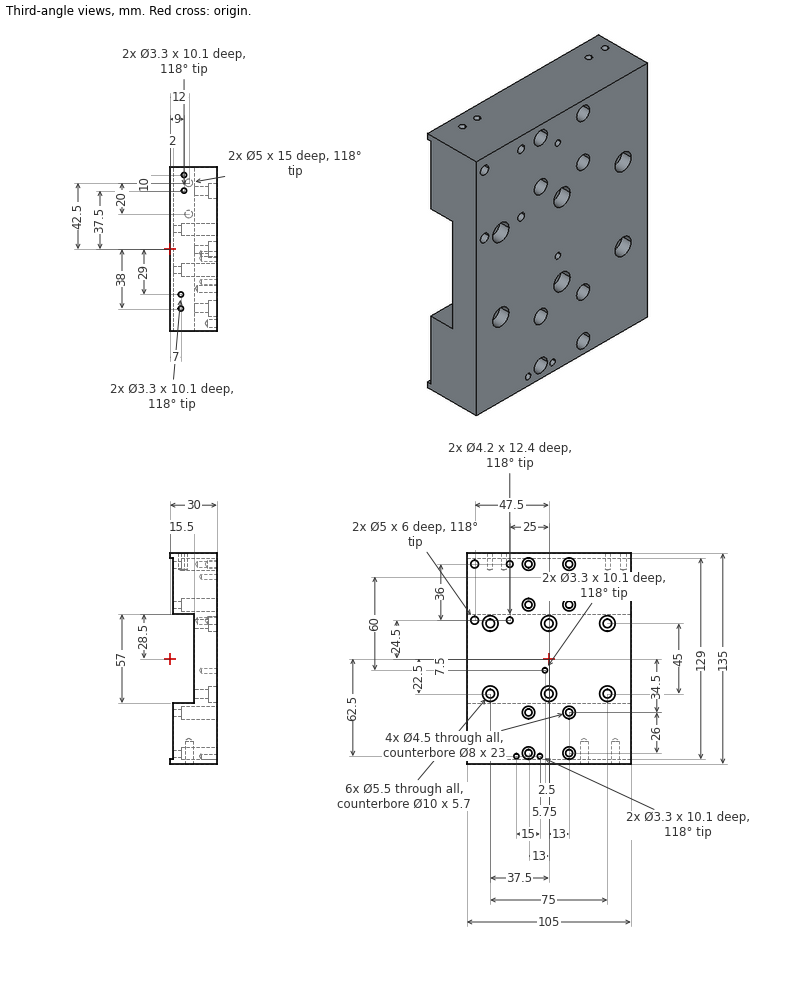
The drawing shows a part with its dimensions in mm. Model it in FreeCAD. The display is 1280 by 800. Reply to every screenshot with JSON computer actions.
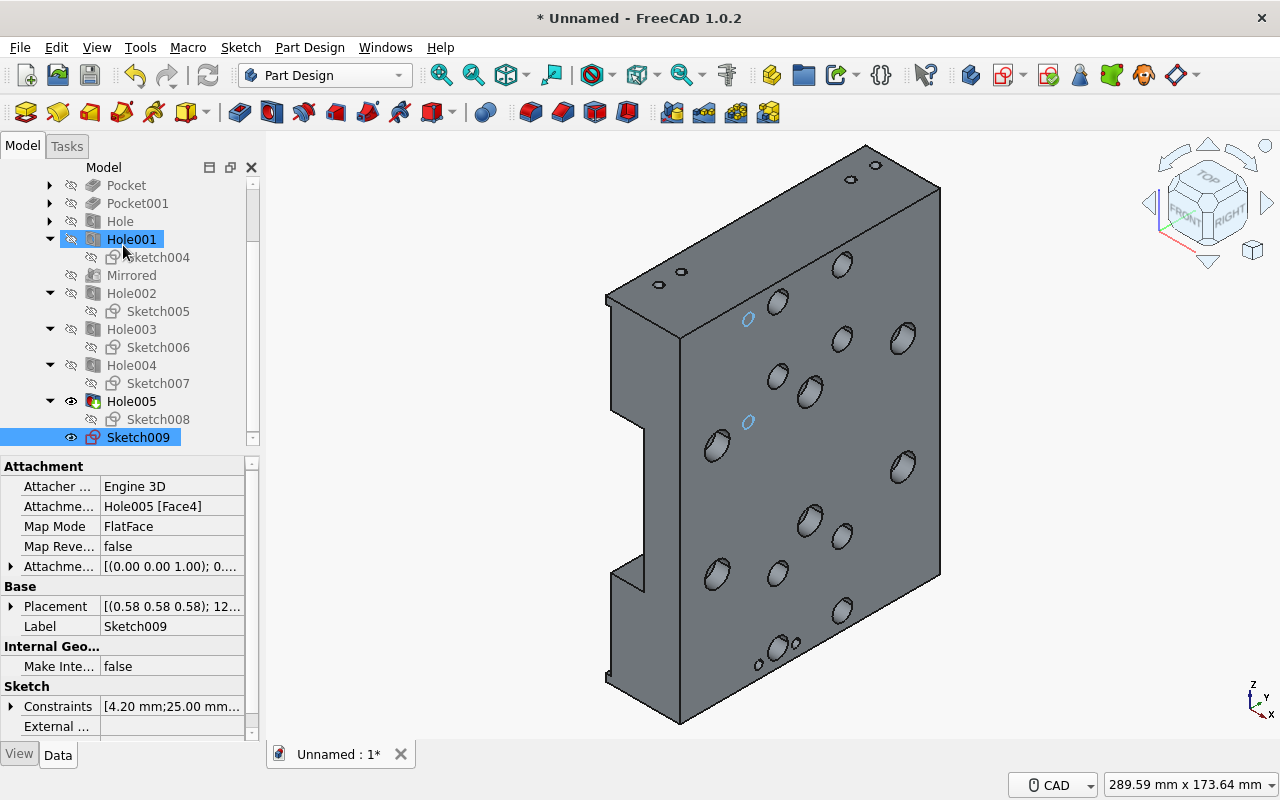
{"action": "left_click", "coordinate": [272, 112]}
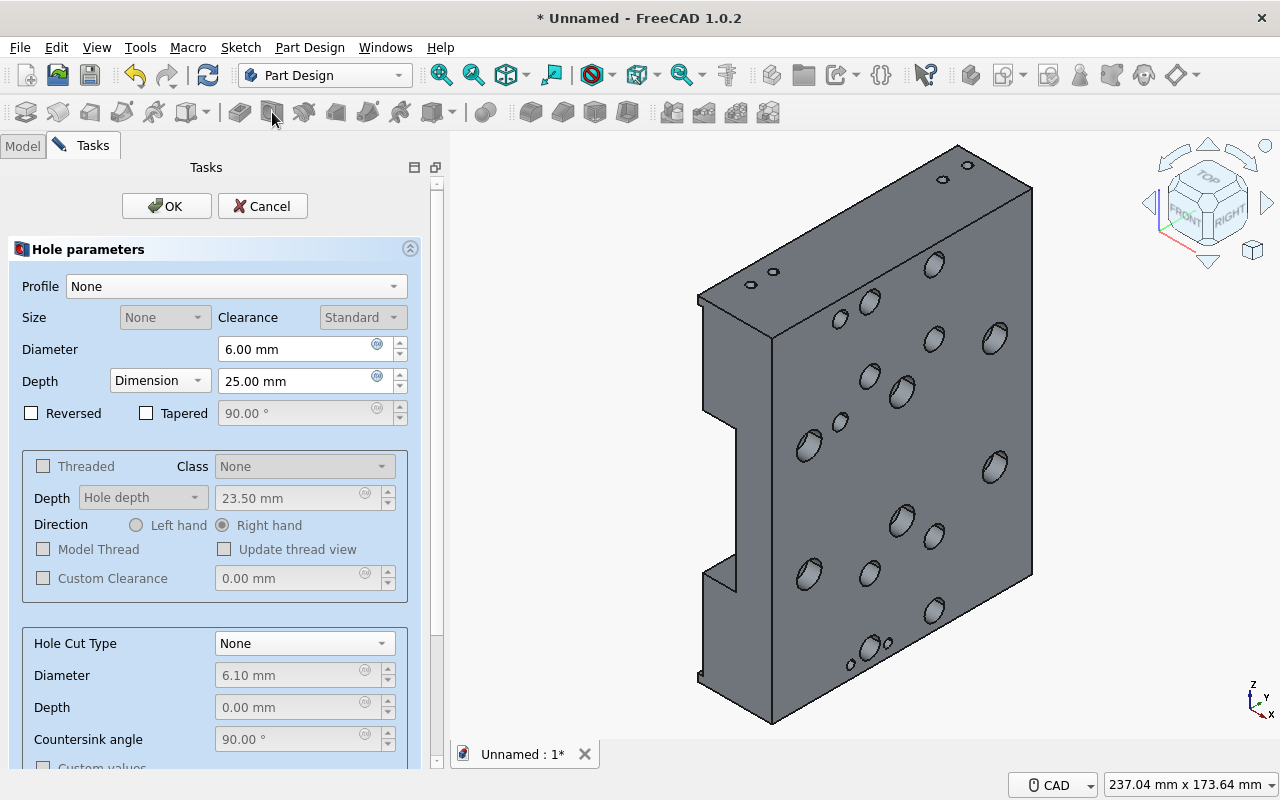
{"action": "triple_click", "coordinate": [305, 349]}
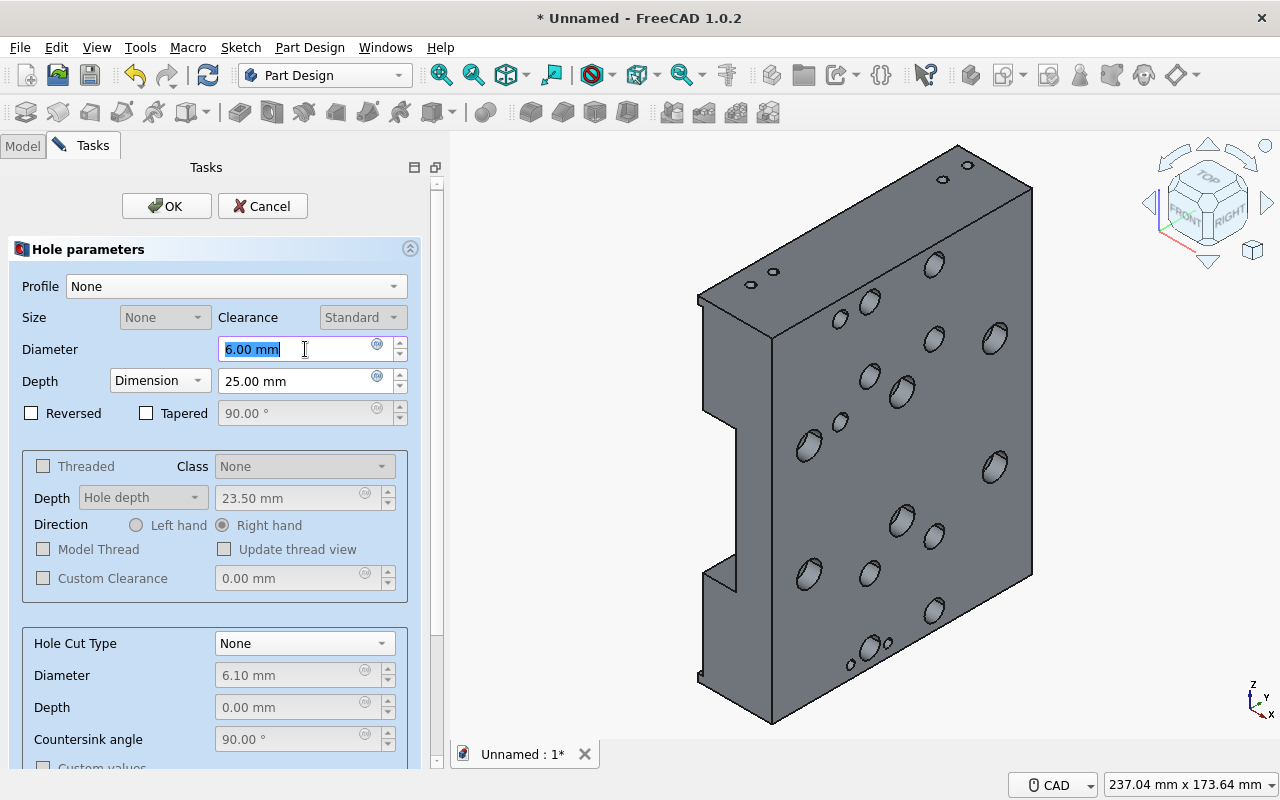
{"action": "type", "text": "4.2"}
{"action": "key", "text": "Tab"}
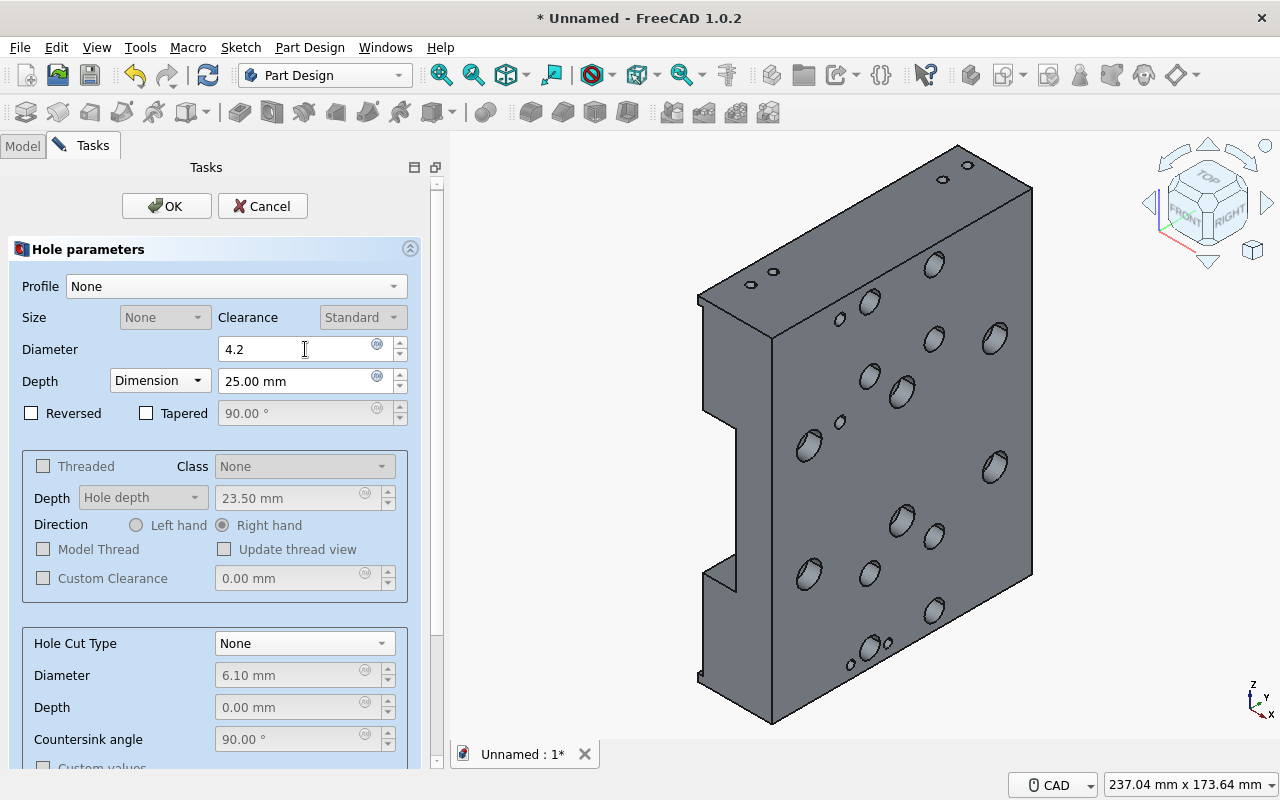
{"action": "triple_click", "coordinate": [305, 381]}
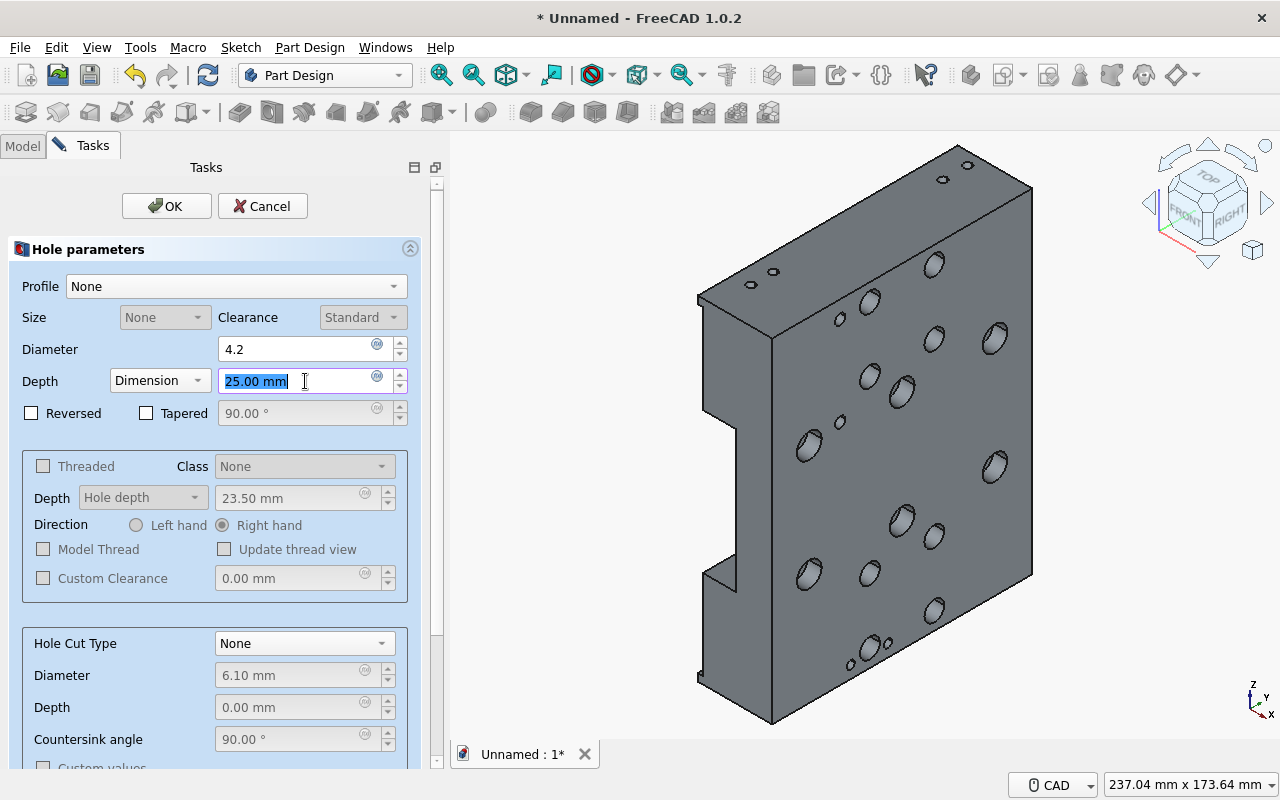
{"action": "type", "text": "12.4"}
{"action": "key", "text": "Tab"}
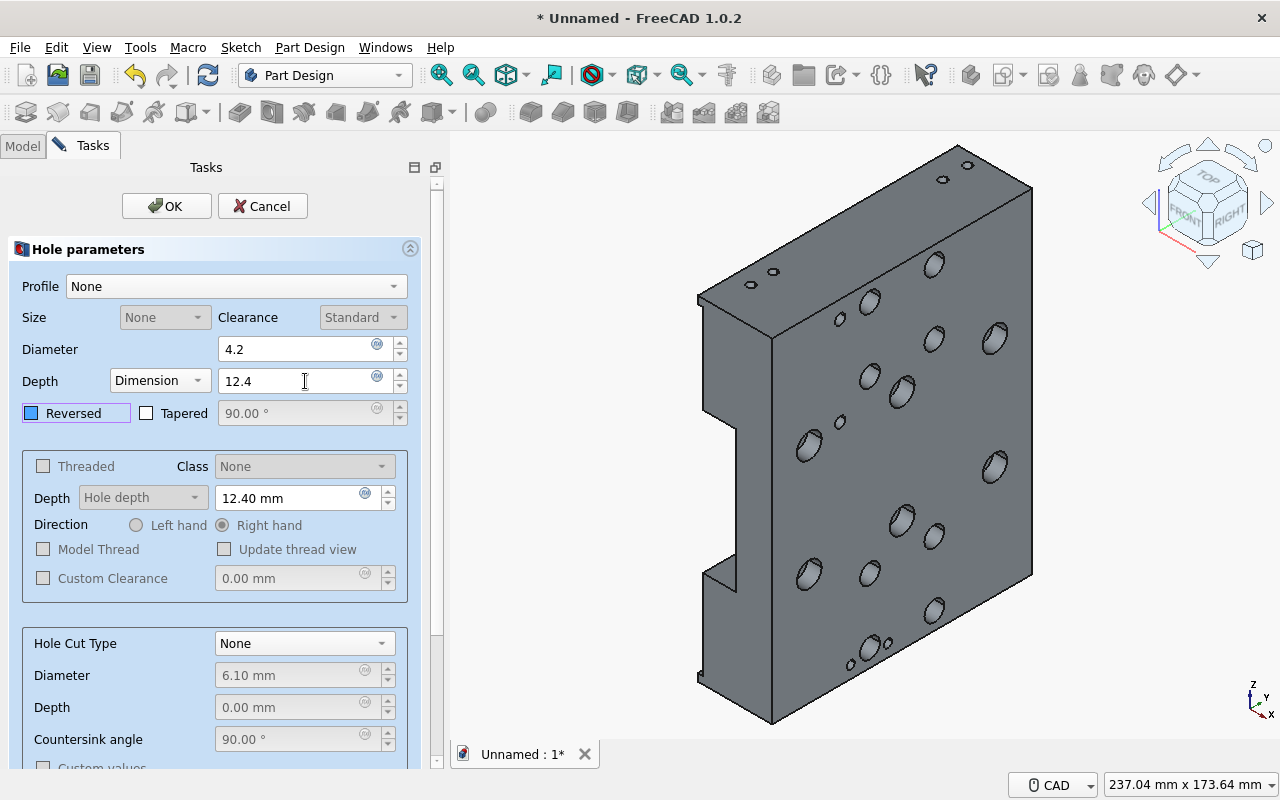
{"action": "left_click", "coordinate": [167, 206]}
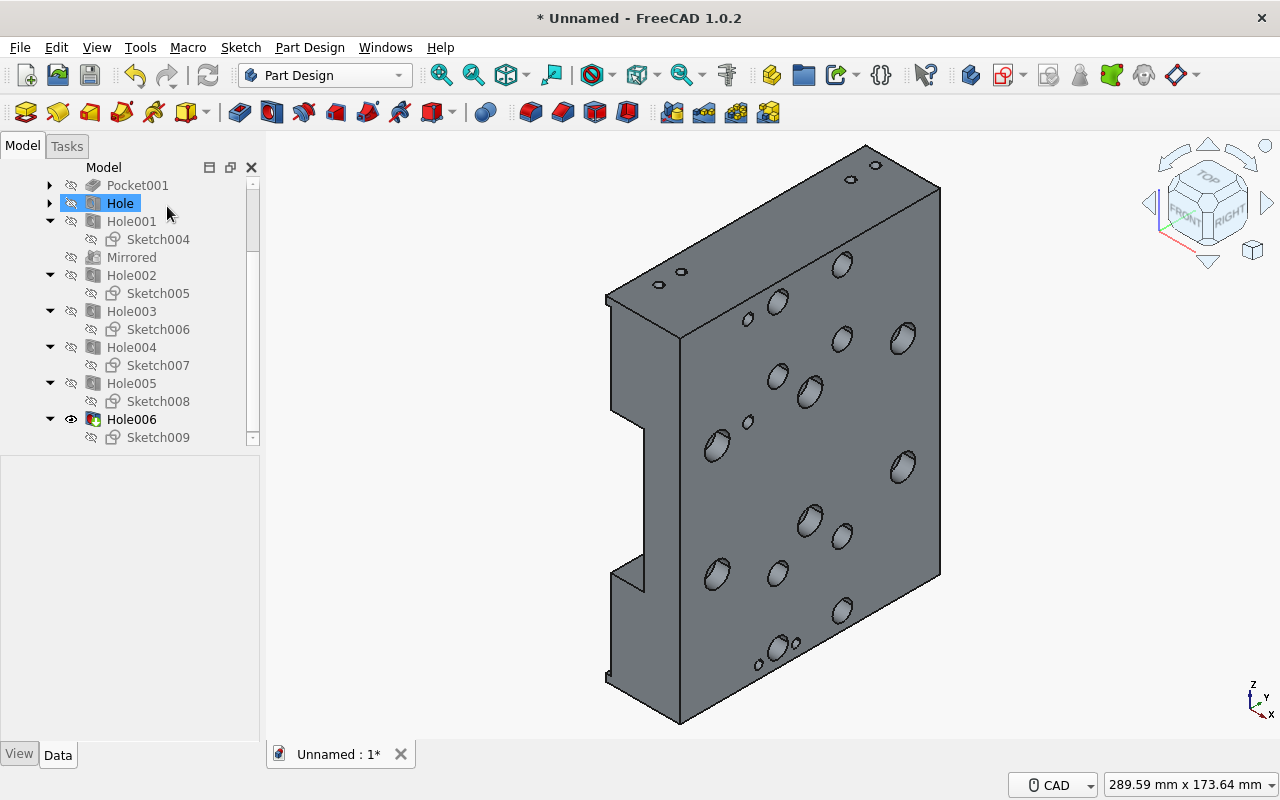
{"action": "left_click", "coordinate": [773, 477]}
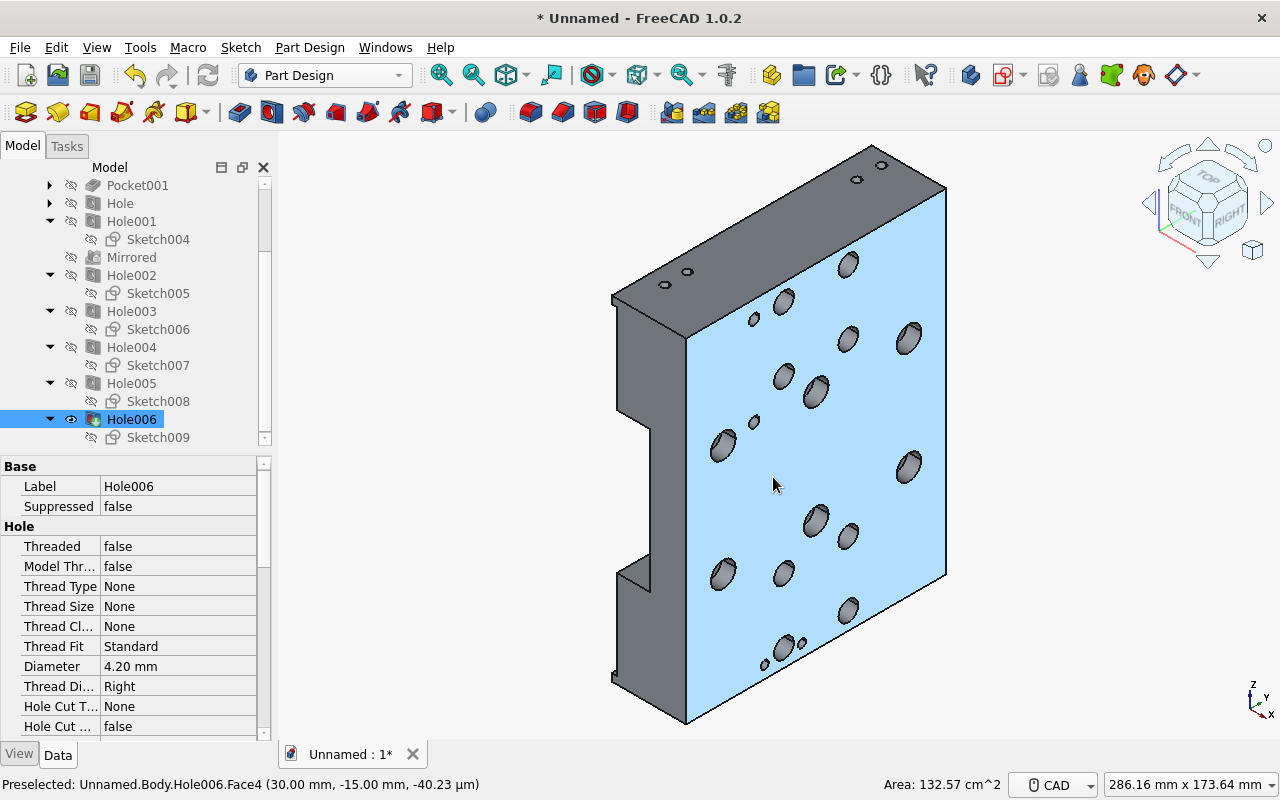
{"action": "left_click", "coordinate": [1004, 76]}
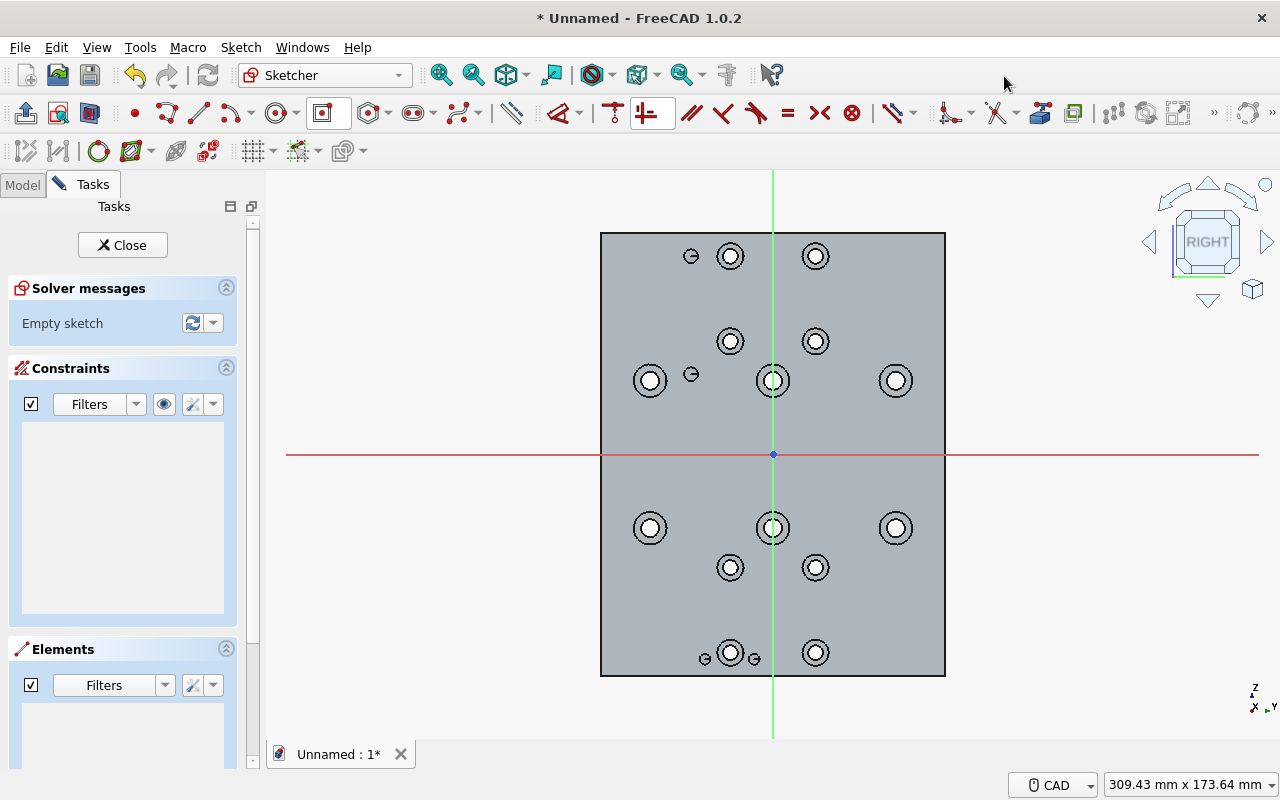
{"action": "scroll", "coordinate": [675, 226], "scroll_direction": "up", "scroll_amount": 3}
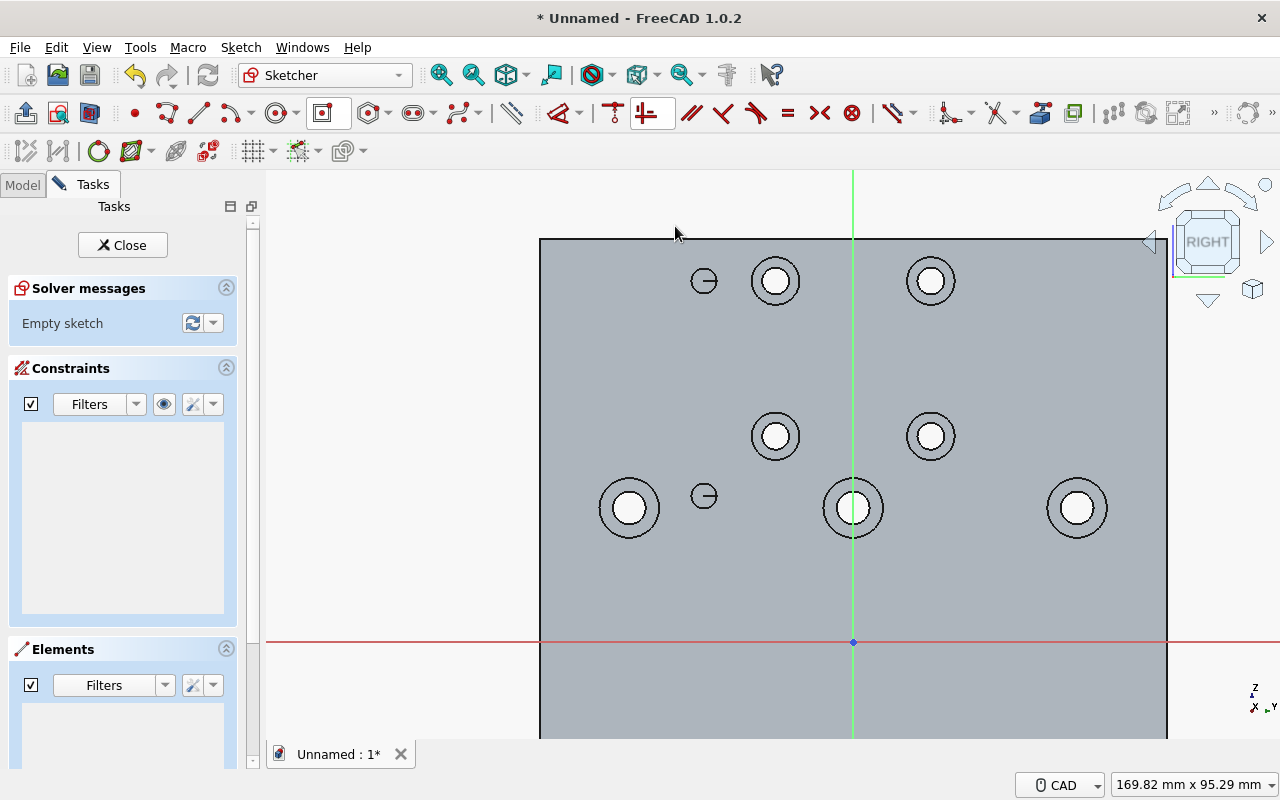
{"action": "left_click", "coordinate": [276, 114]}